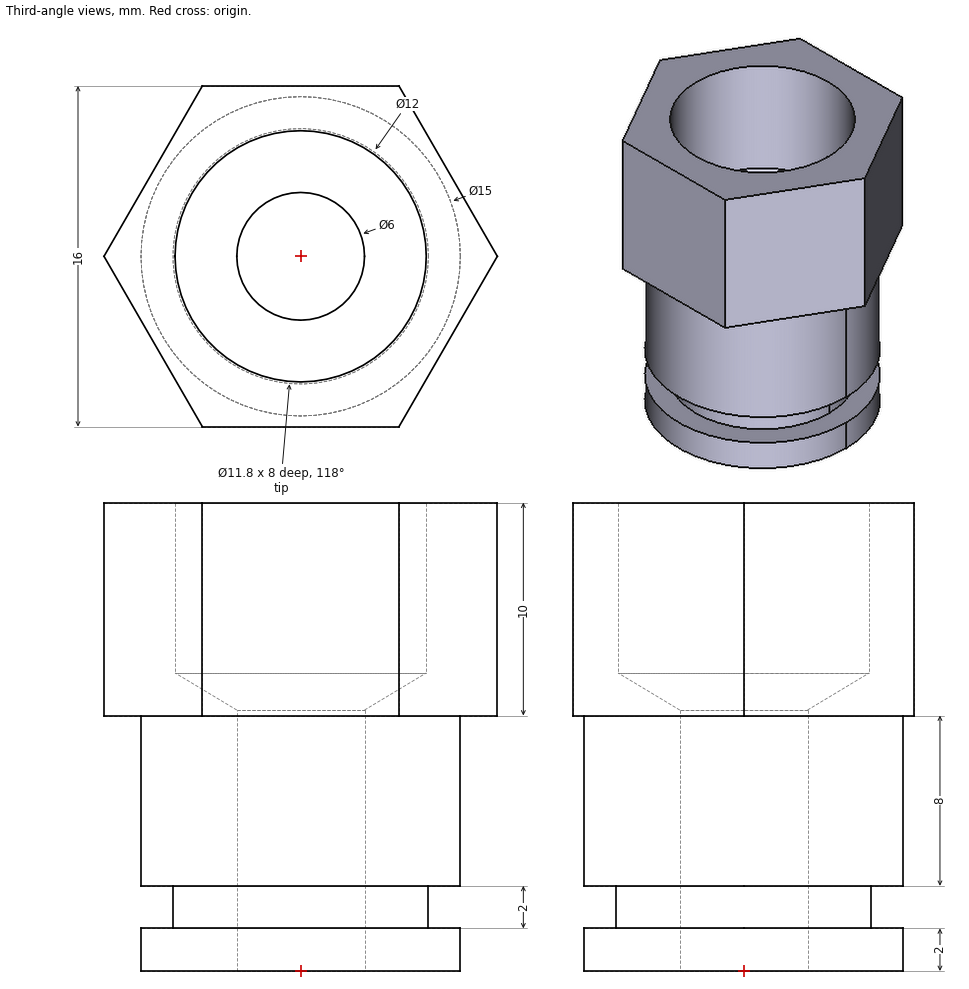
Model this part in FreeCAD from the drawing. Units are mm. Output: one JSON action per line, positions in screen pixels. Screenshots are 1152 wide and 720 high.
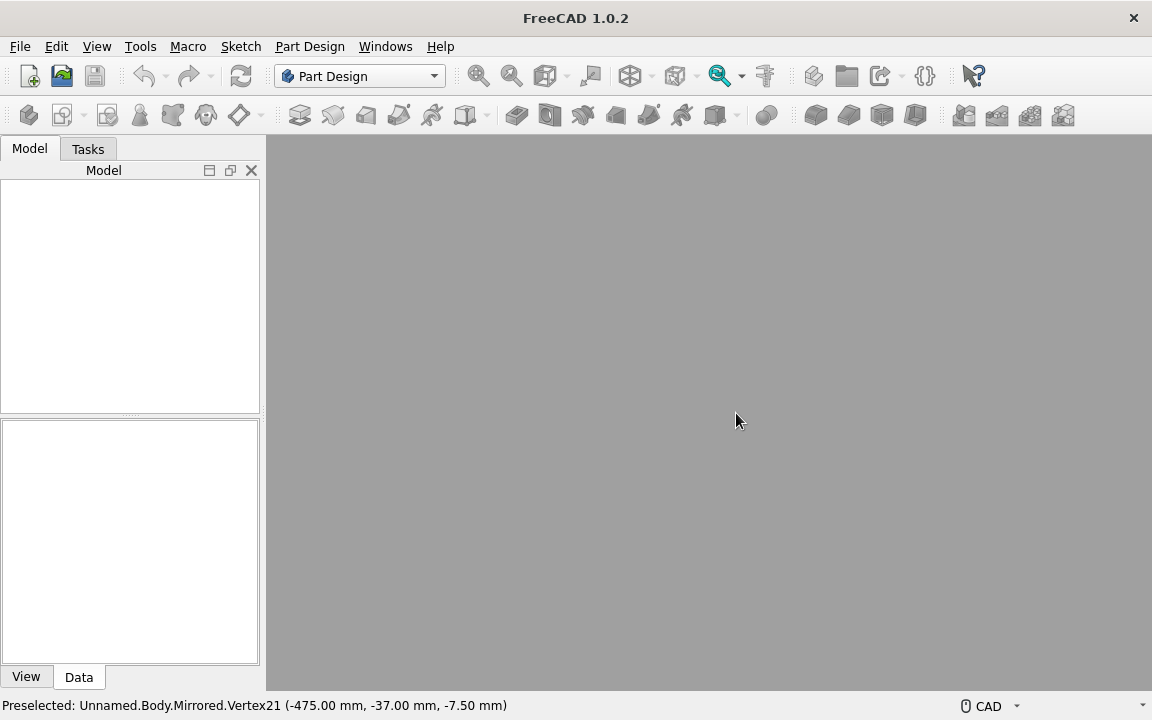
{"action": "key", "text": "ctrl+n"}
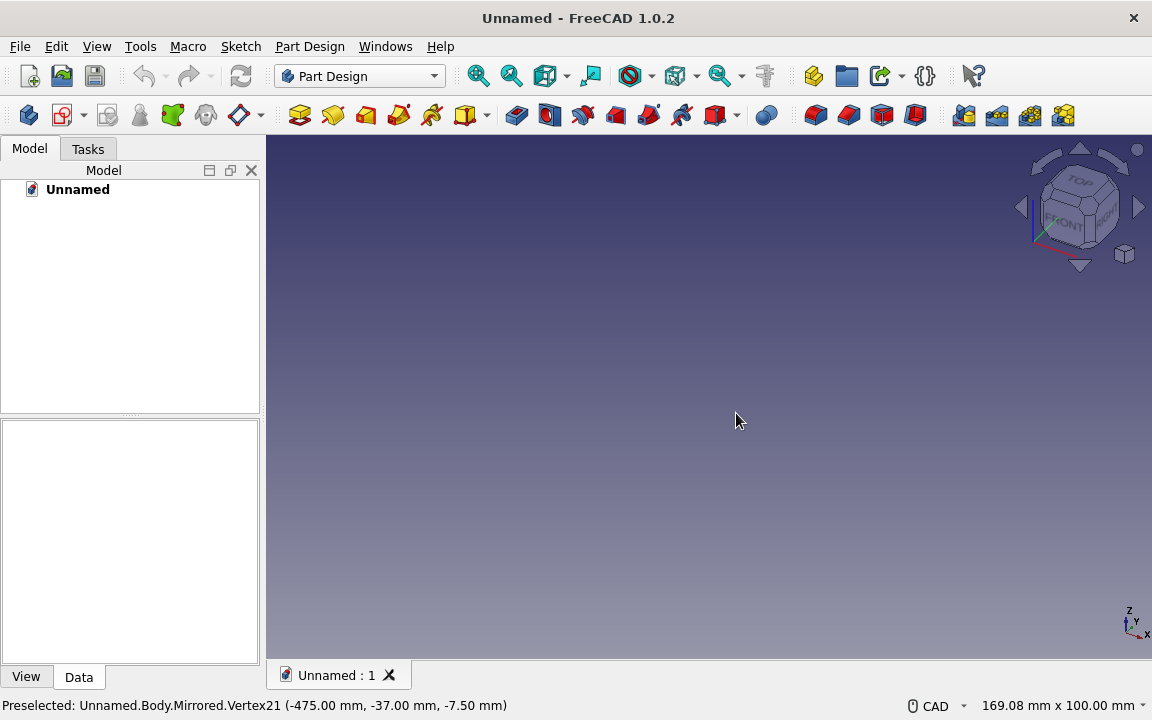
{"action": "left_click", "coordinate": [62, 116]}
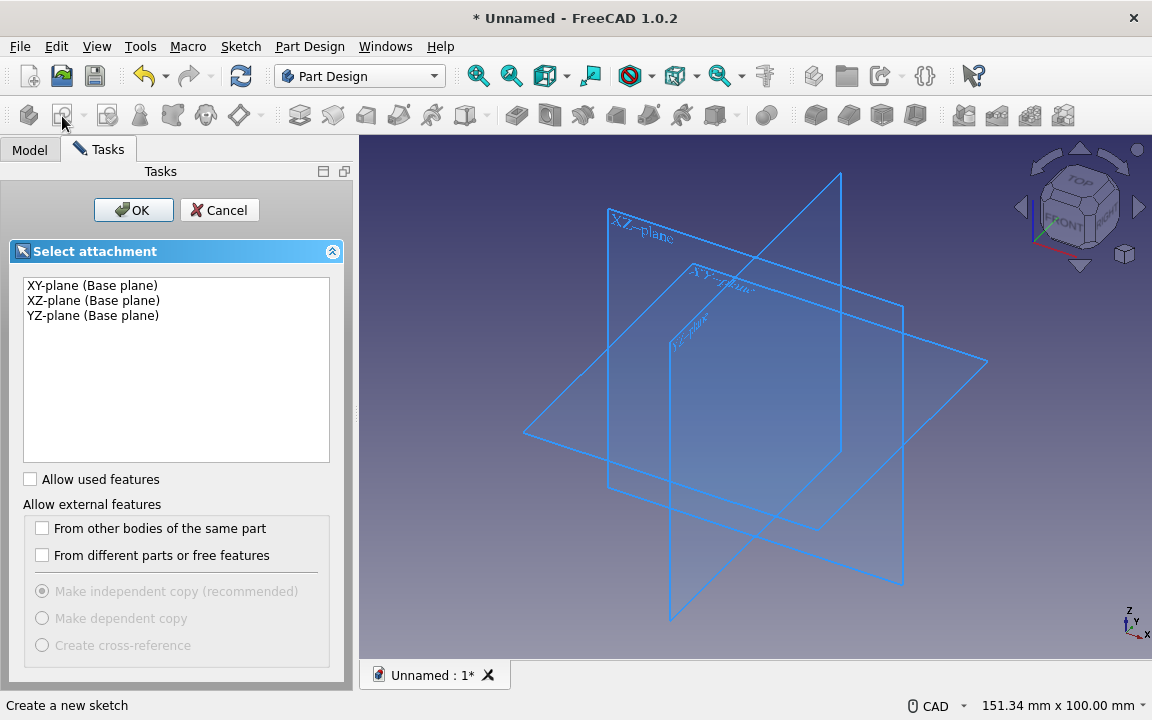
{"action": "left_click", "coordinate": [84, 286]}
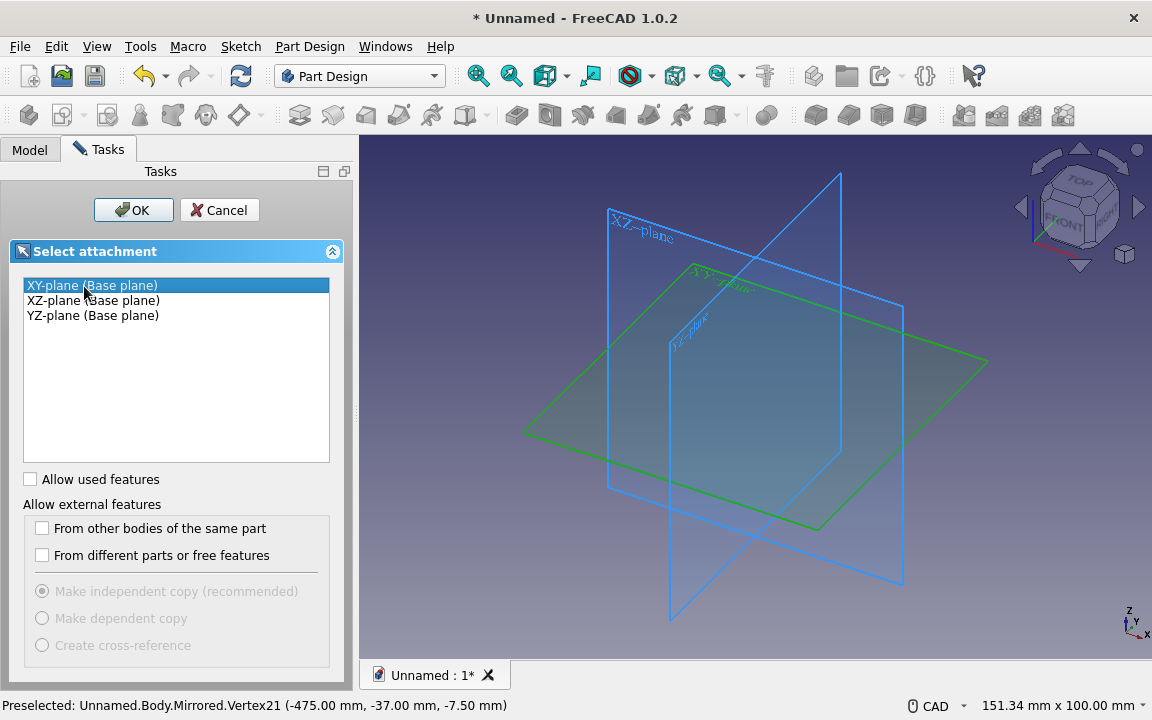
{"action": "left_click", "coordinate": [134, 210]}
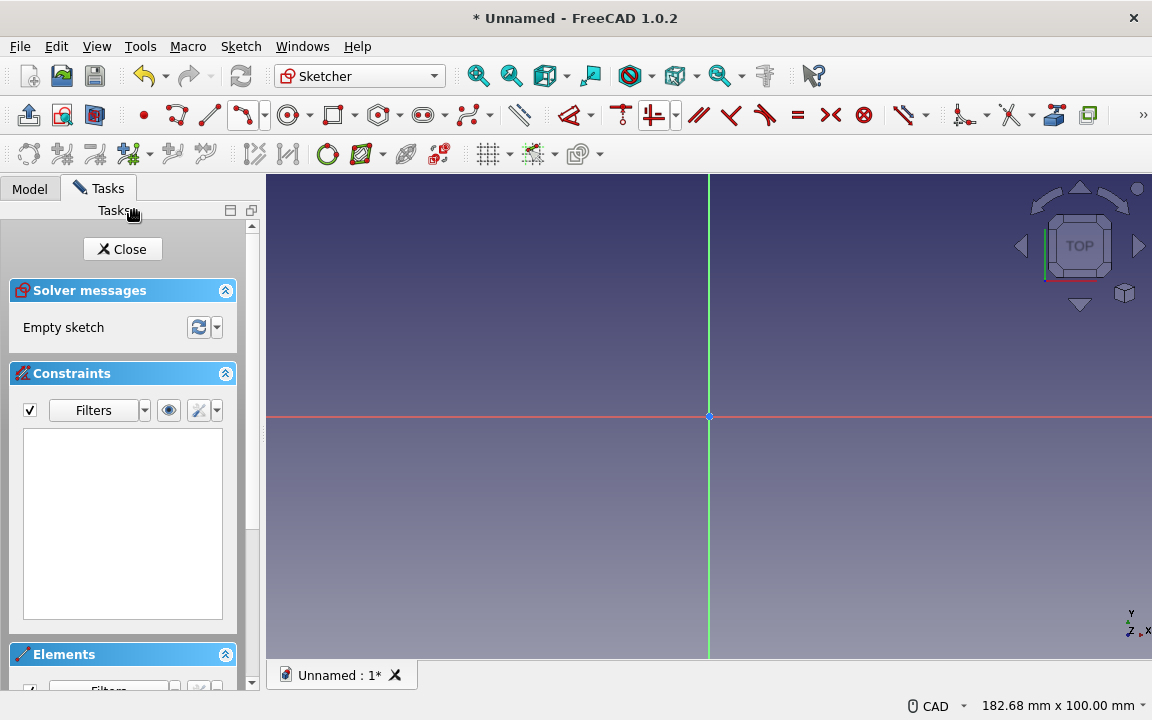
{"action": "scroll", "coordinate": [731, 416], "scroll_direction": "up", "scroll_amount": 7}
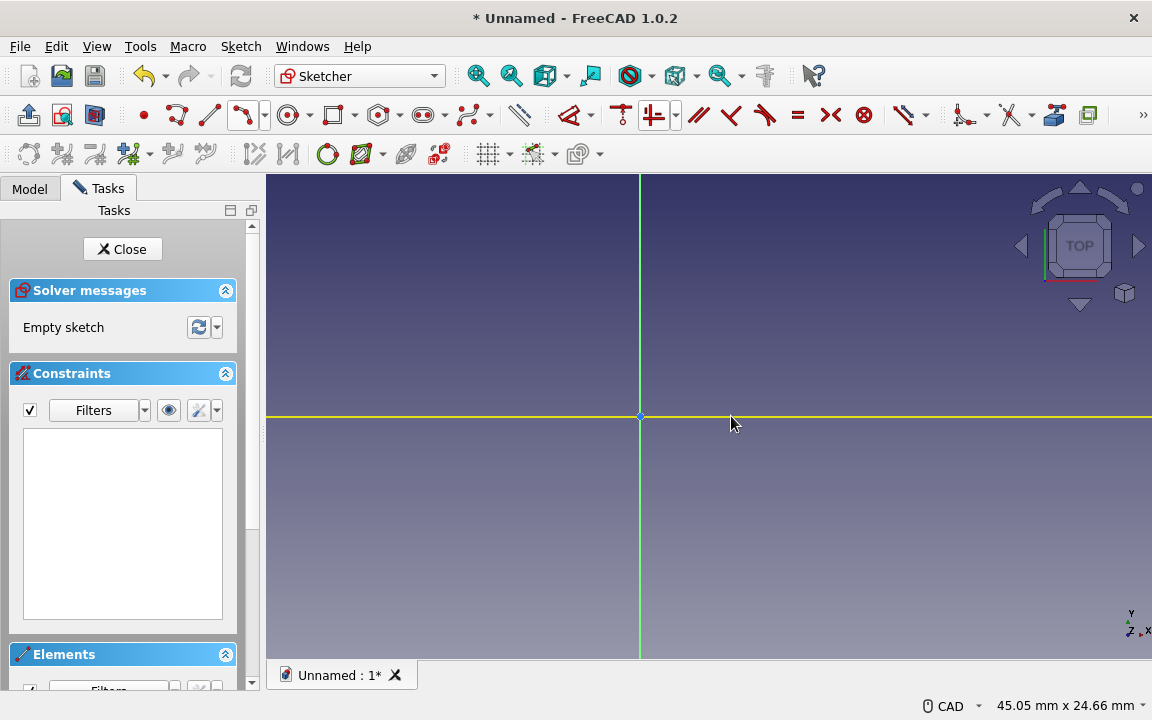
{"action": "left_click", "coordinate": [288, 116]}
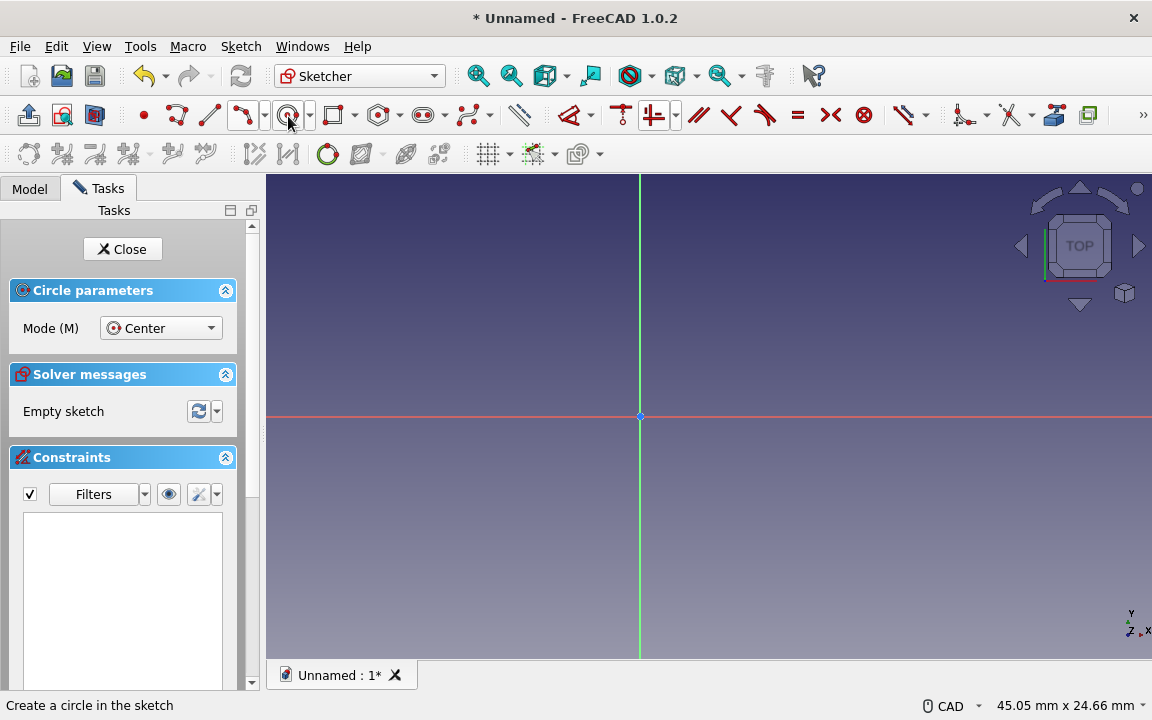
{"action": "left_click", "coordinate": [640, 416]}
{"action": "left_click", "coordinate": [744, 312]}
{"action": "key", "text": "Escape"}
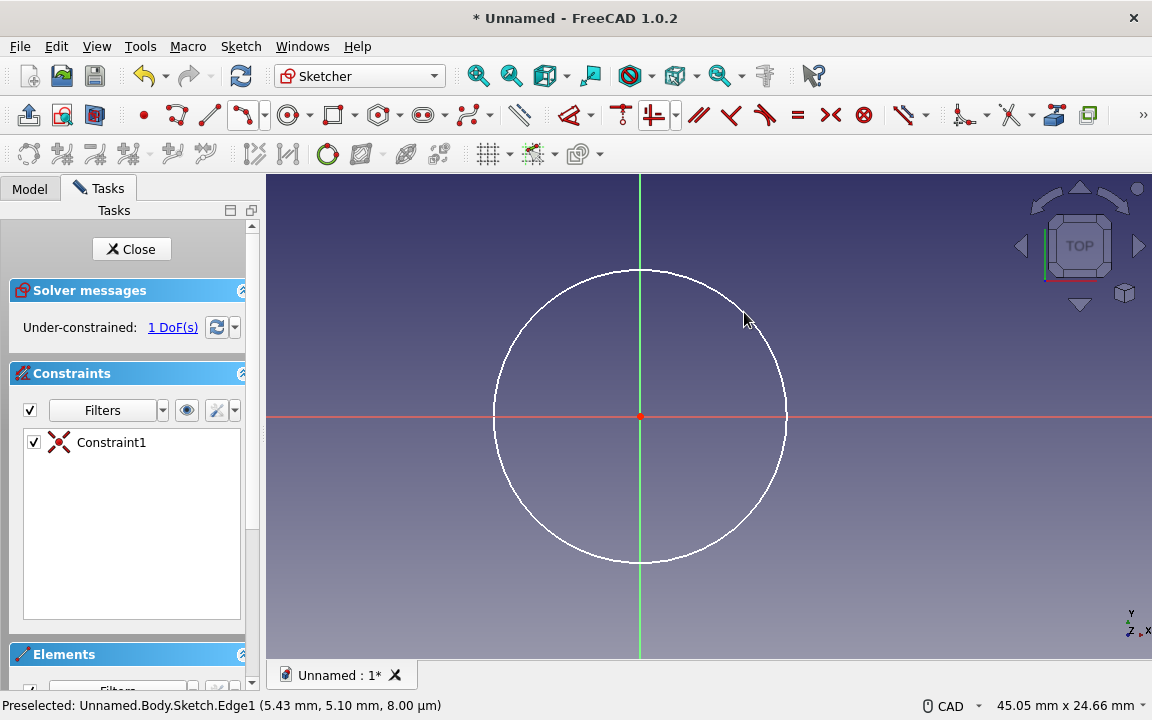
{"action": "key", "text": "d"}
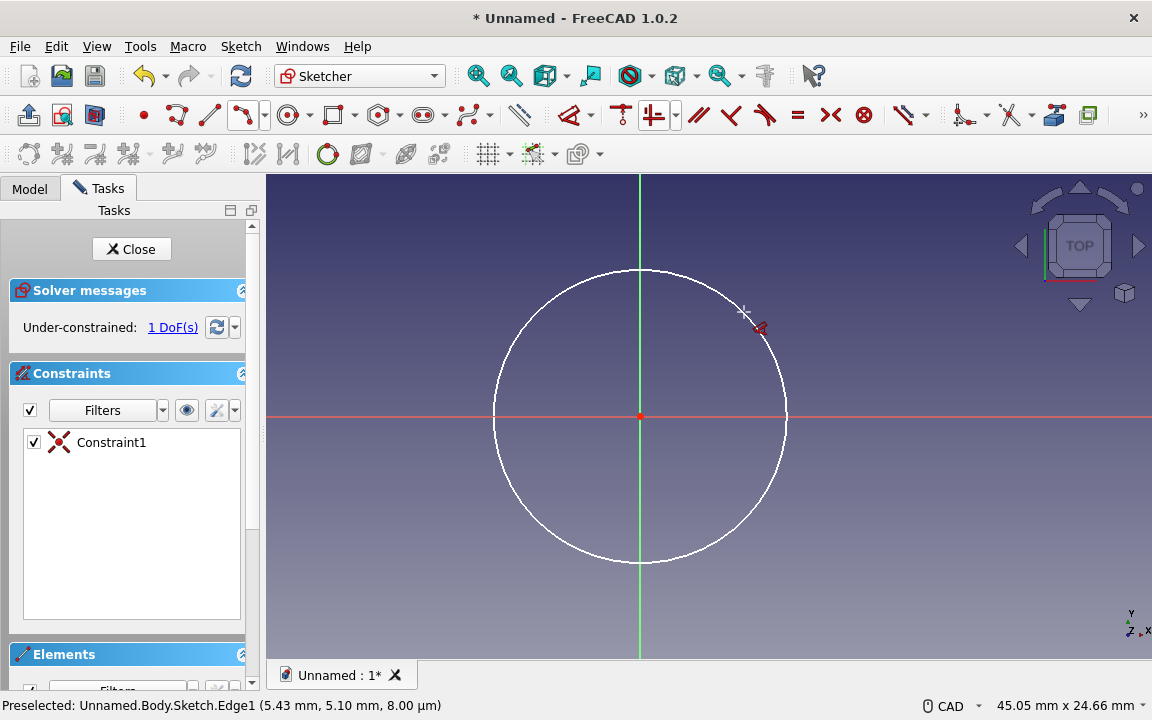
{"action": "left_click", "coordinate": [744, 313]}
{"action": "left_click", "coordinate": [767, 290]}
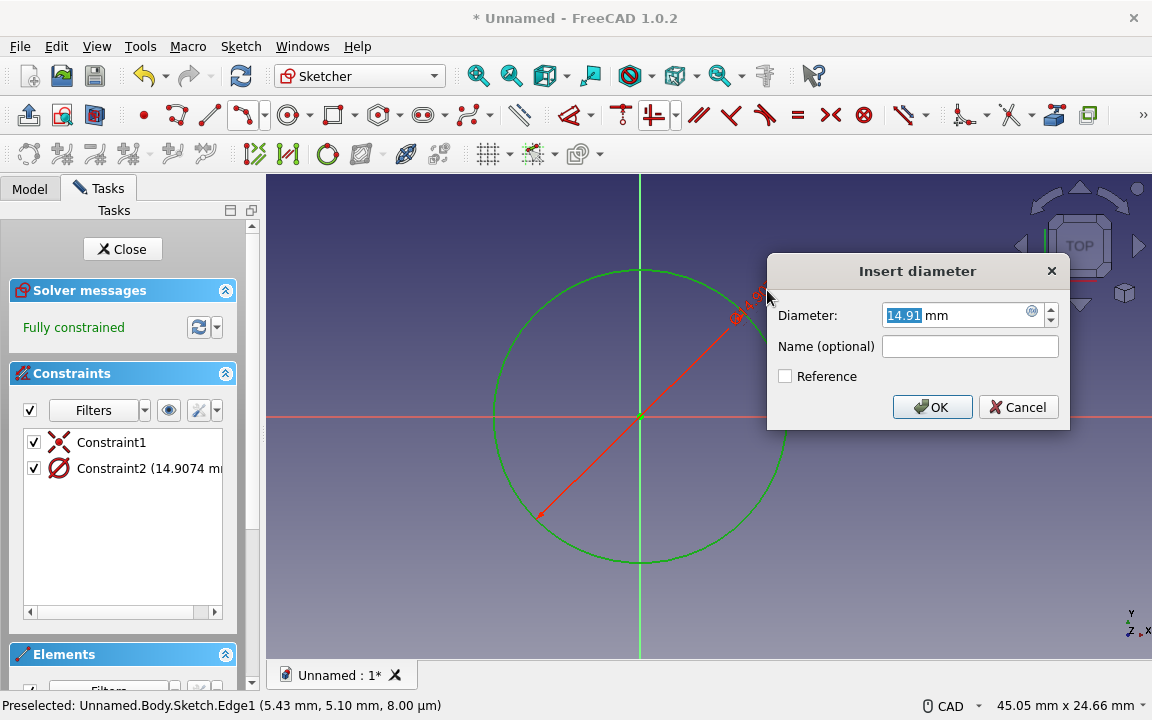
{"action": "type", "text": "15"}
{"action": "key", "text": "Return"}
{"action": "key", "text": "Escape"}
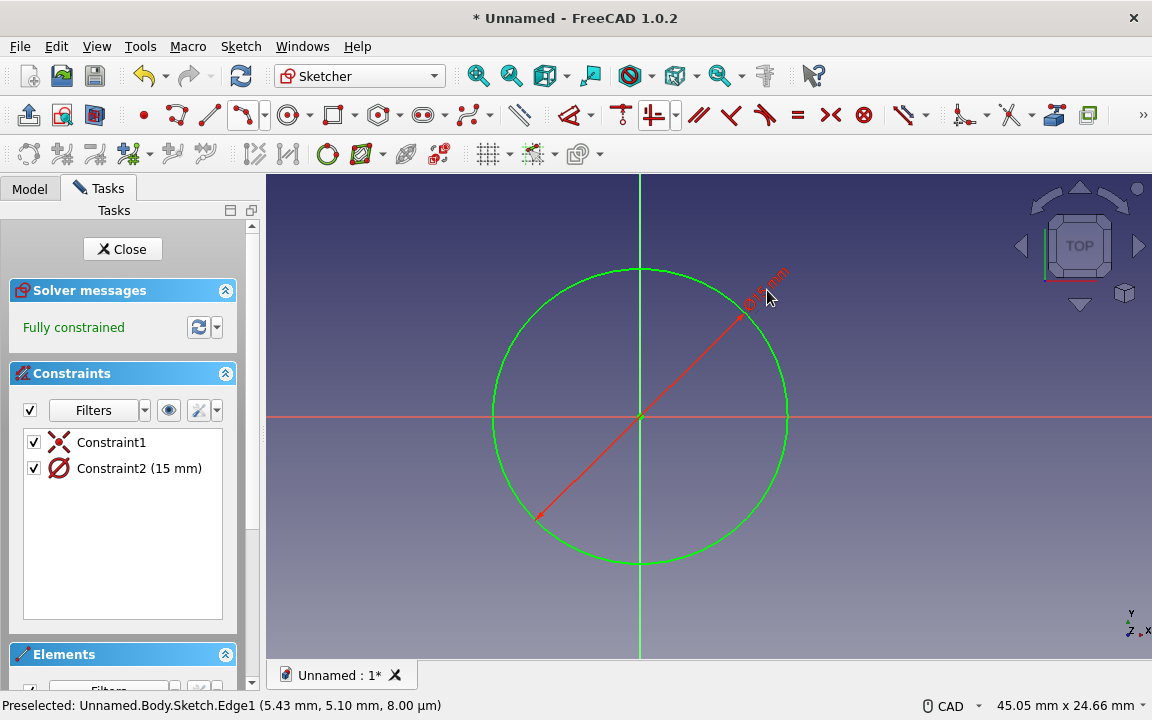
{"action": "left_click", "coordinate": [123, 249]}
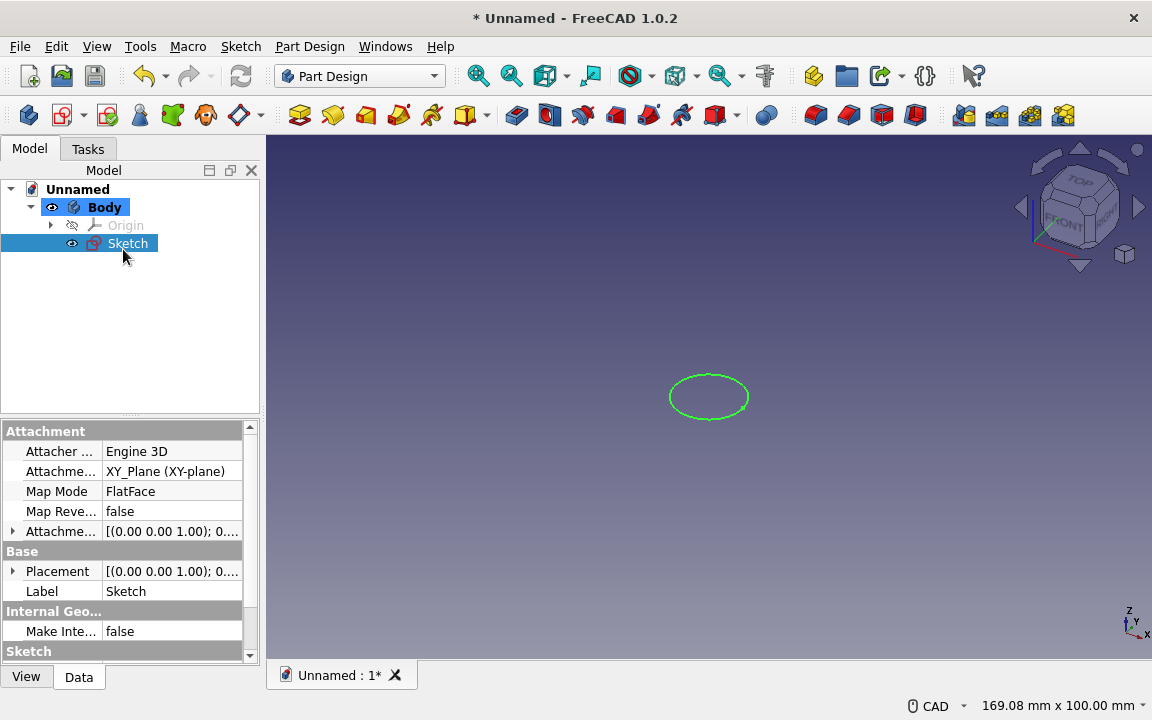
{"action": "left_click", "coordinate": [300, 116]}